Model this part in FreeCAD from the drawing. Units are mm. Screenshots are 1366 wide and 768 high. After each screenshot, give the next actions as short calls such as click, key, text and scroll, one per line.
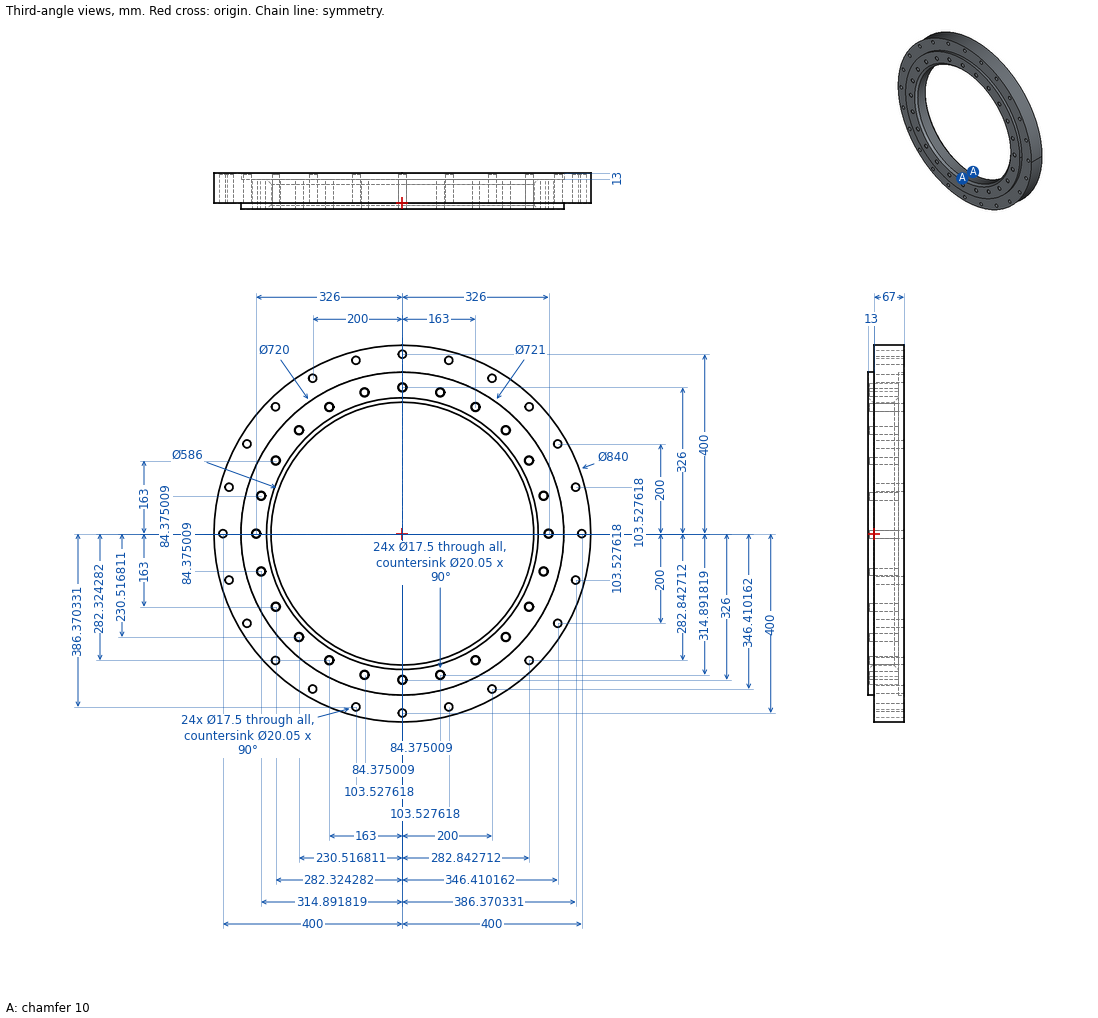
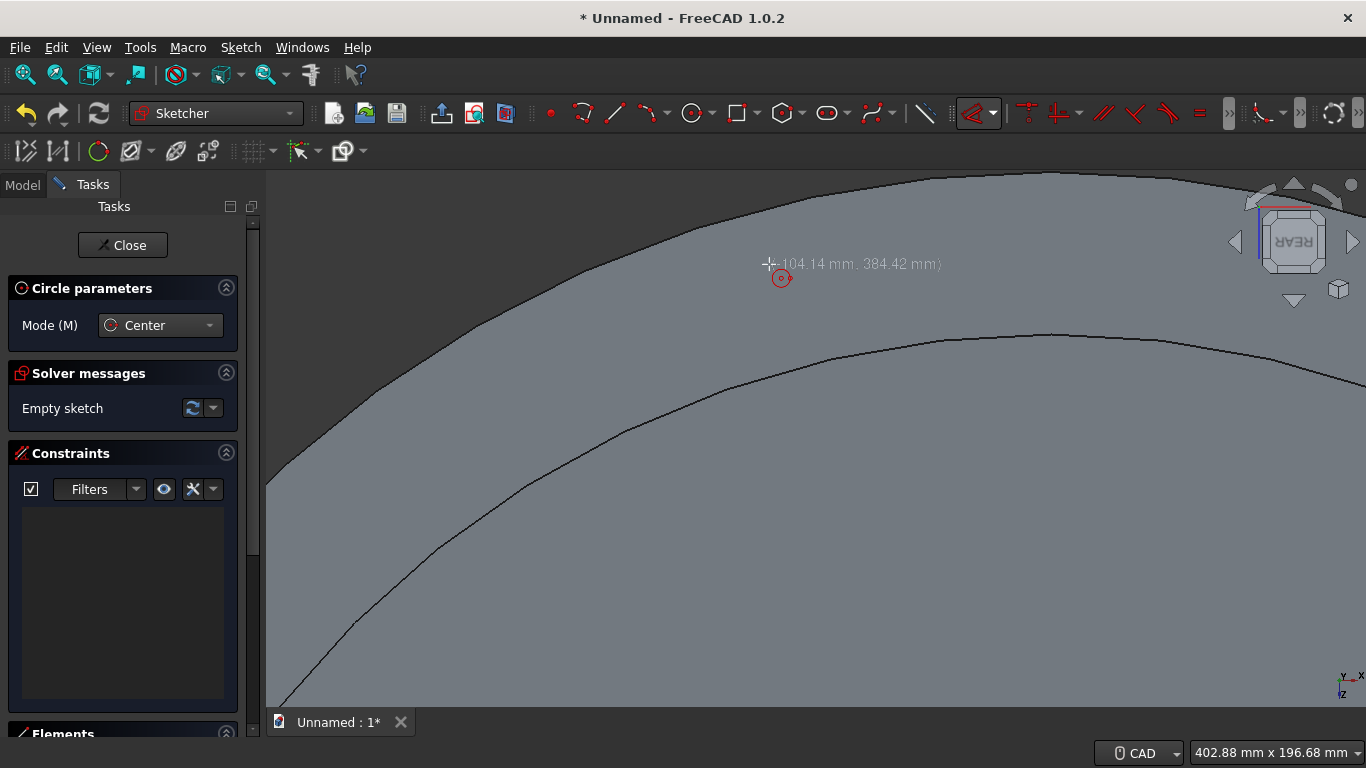
scroll(687, 264, down, 9)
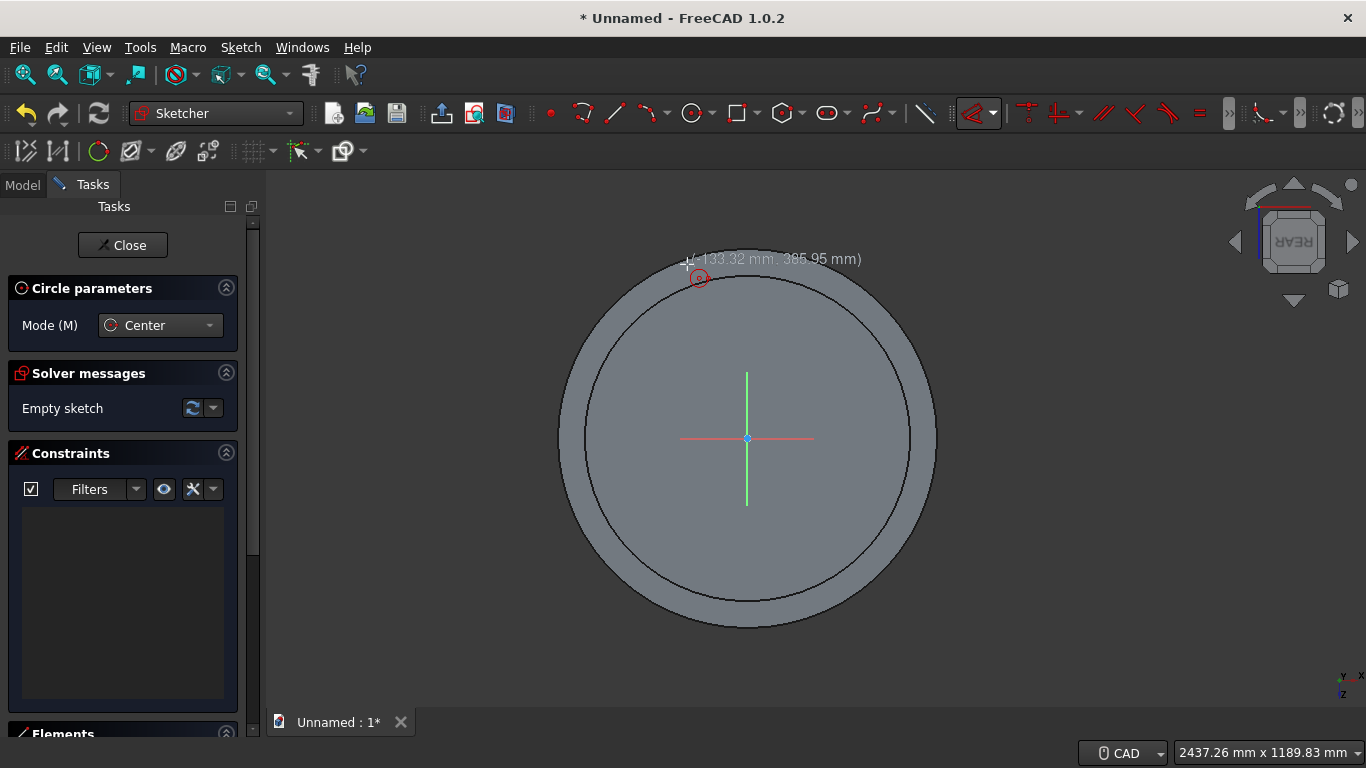
click(701, 264)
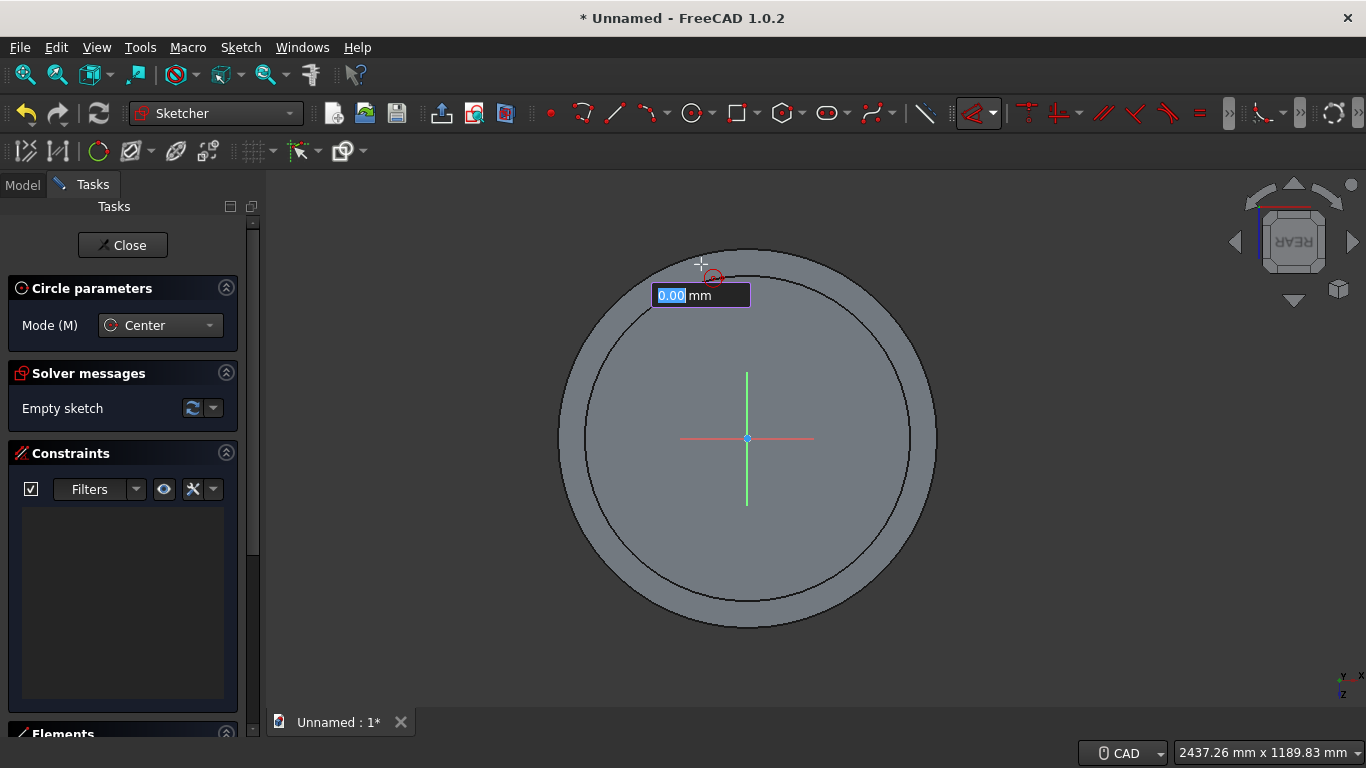
scroll(704, 261, up, 7)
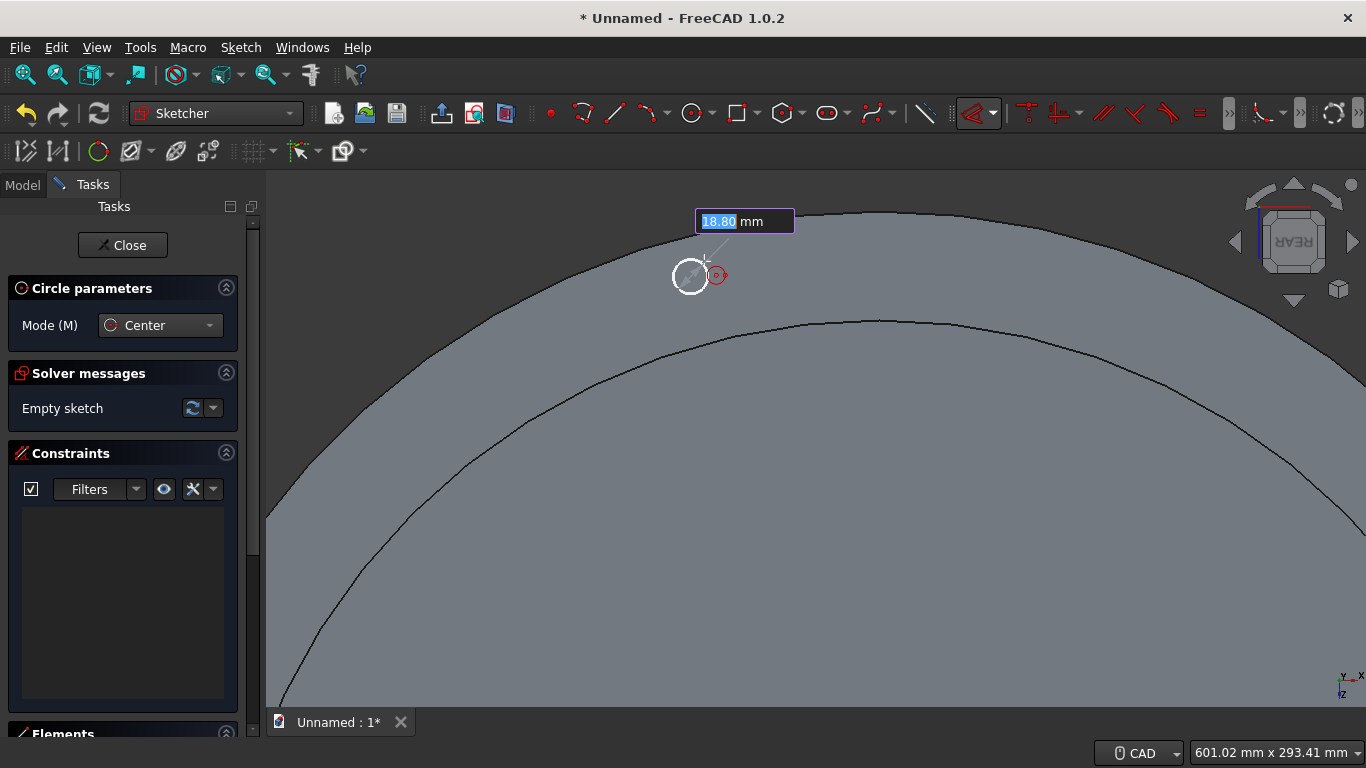
click(701, 262)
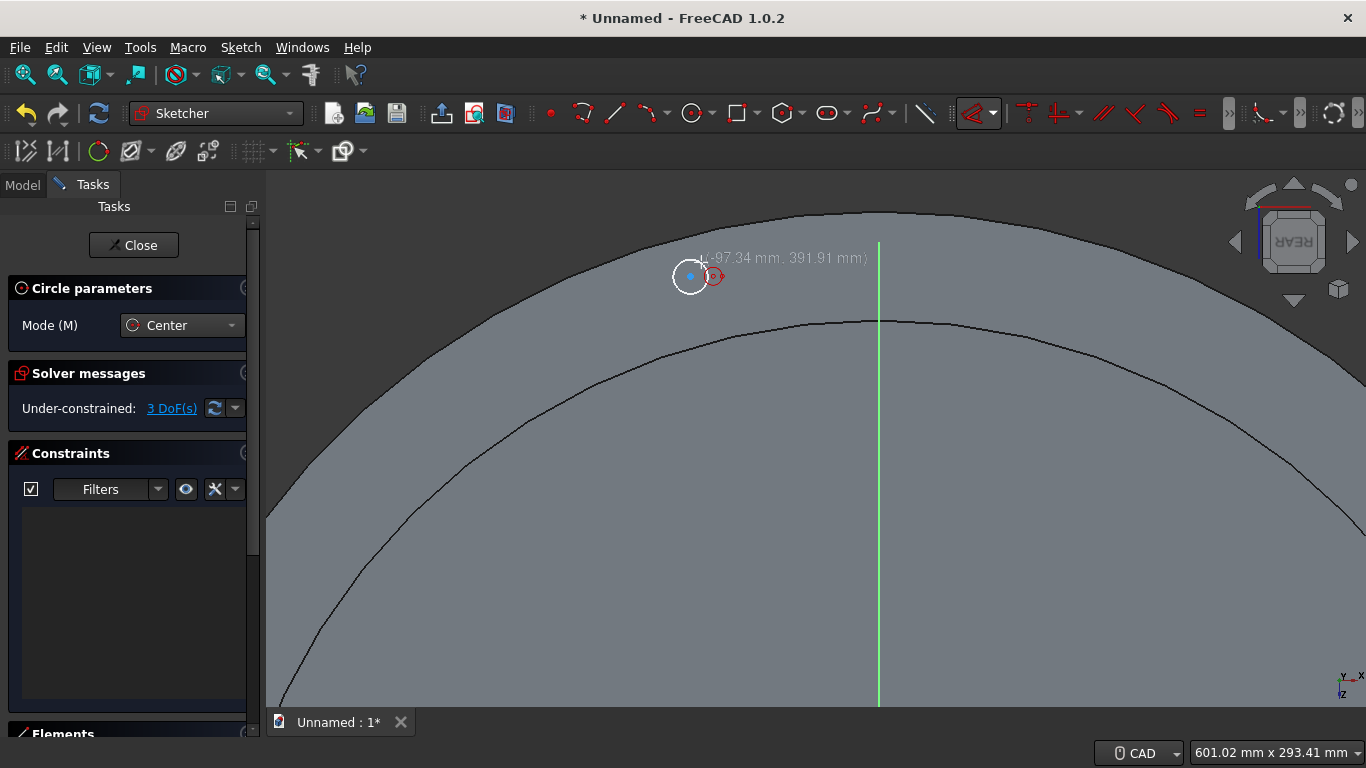
scroll(879, 248, up, 2)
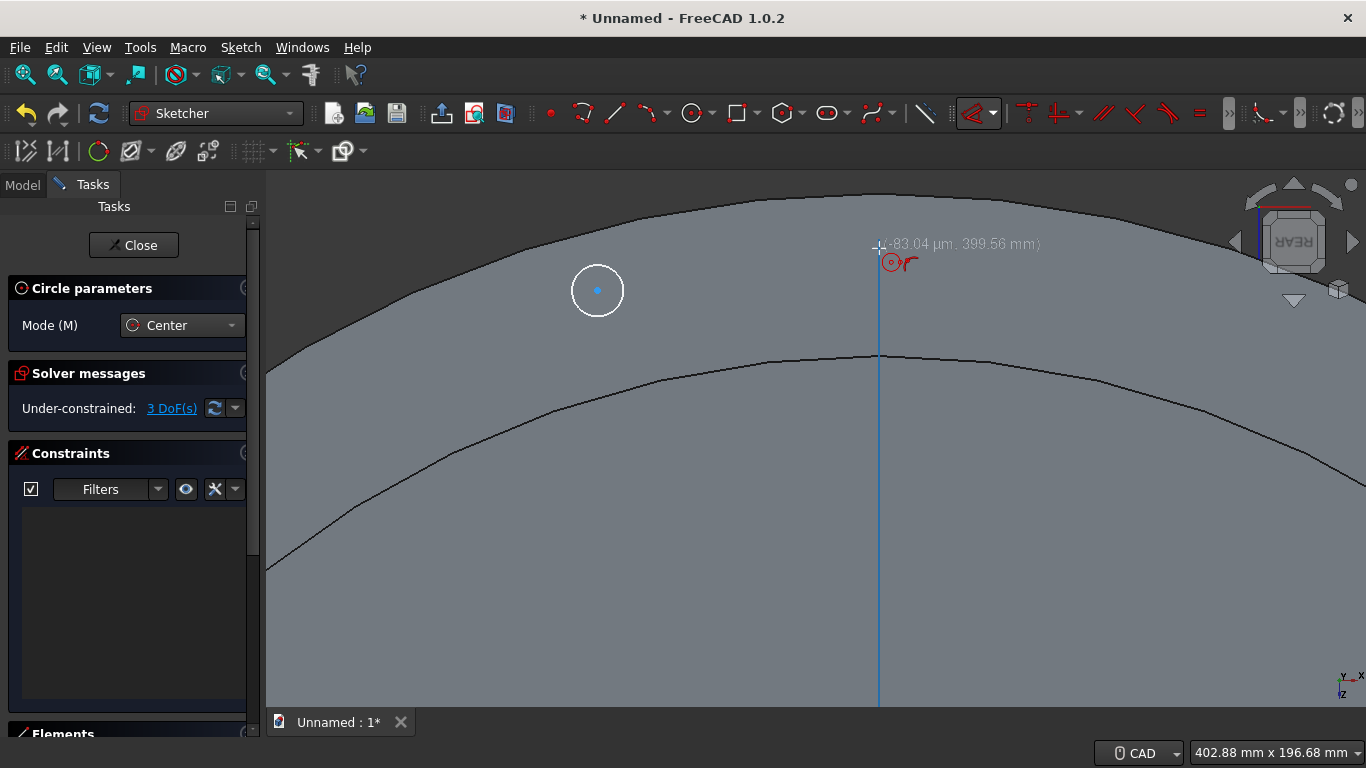
scroll(721, 260, down, 9)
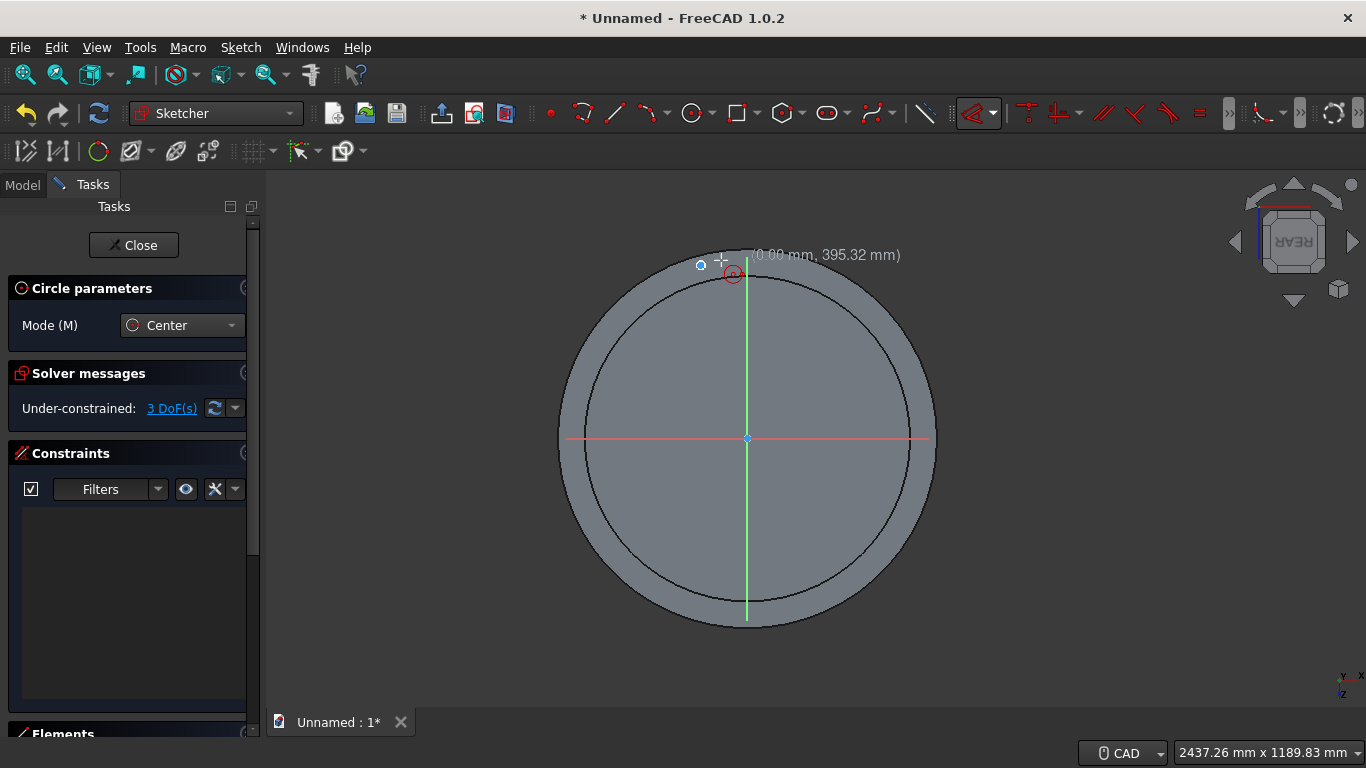
click(747, 258)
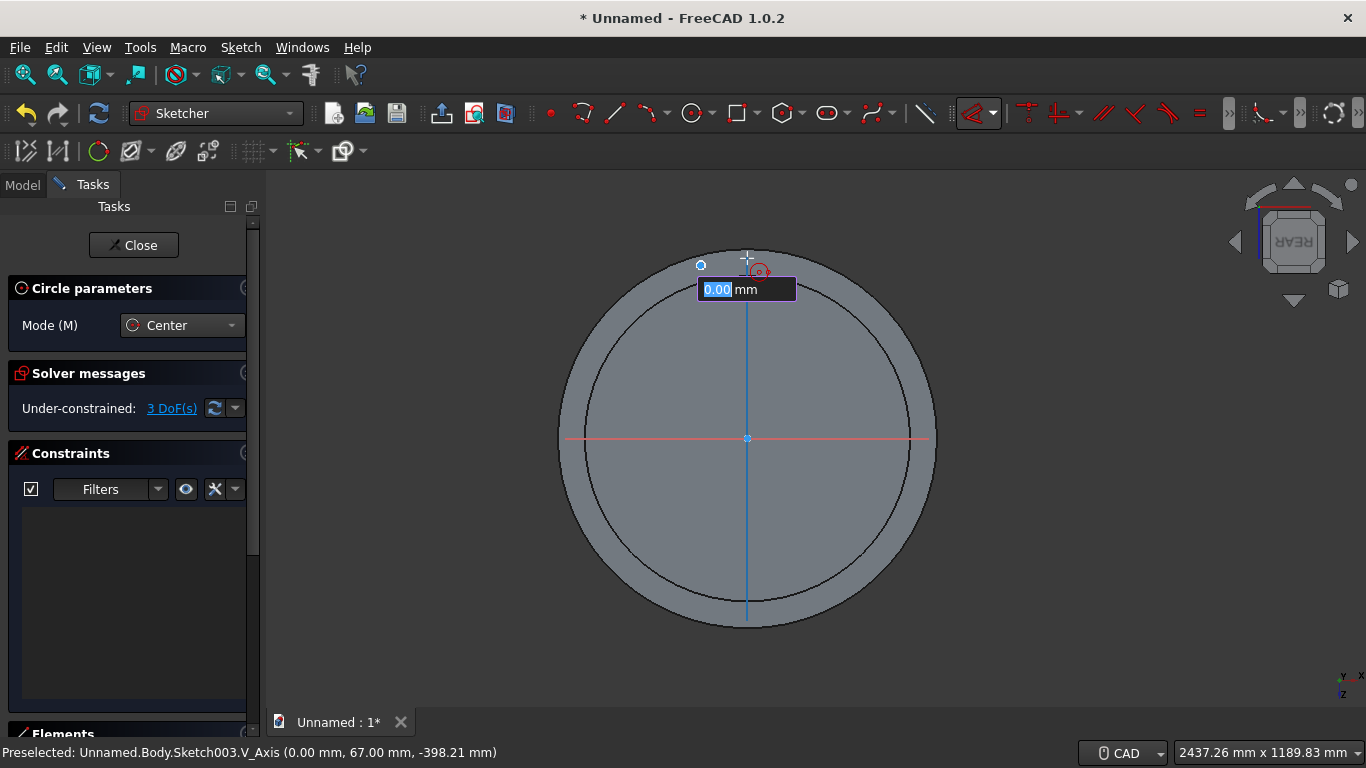
scroll(751, 257, up, 8)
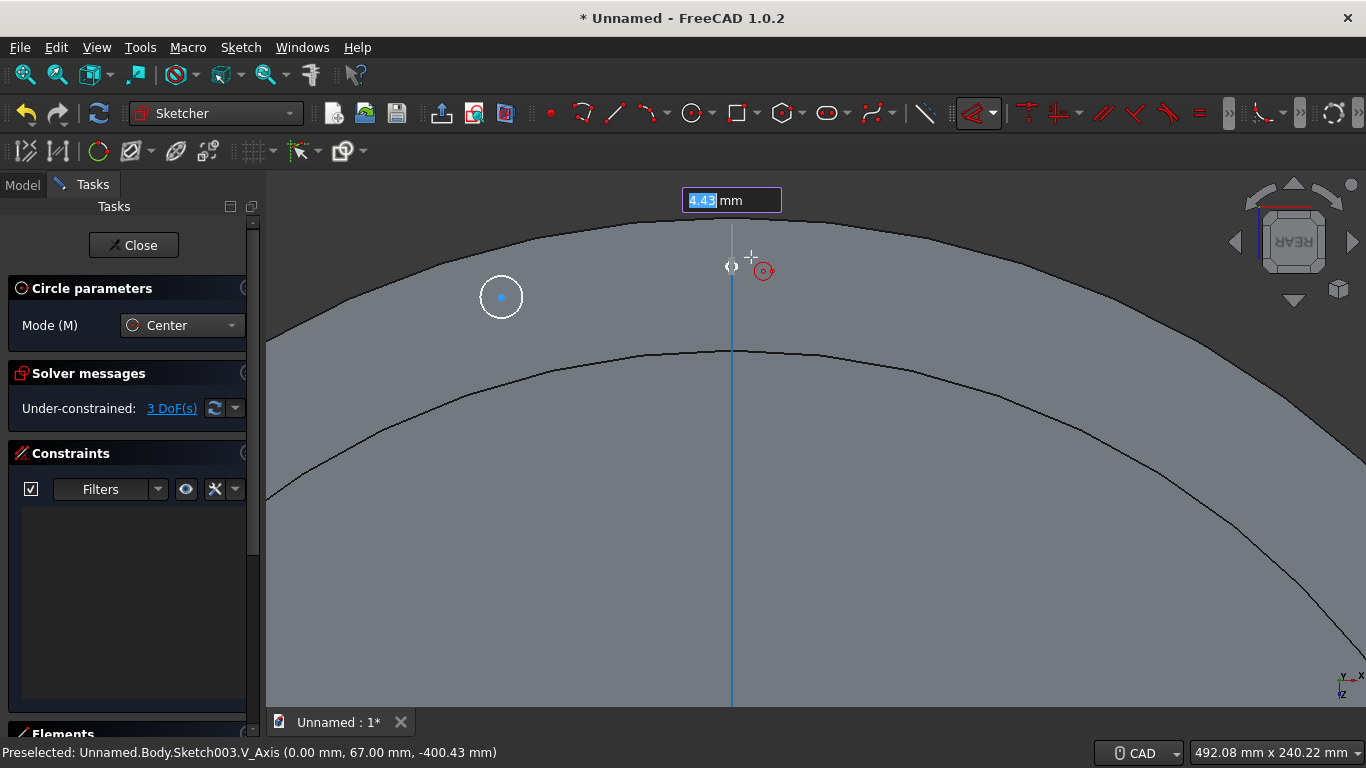
click(750, 256)